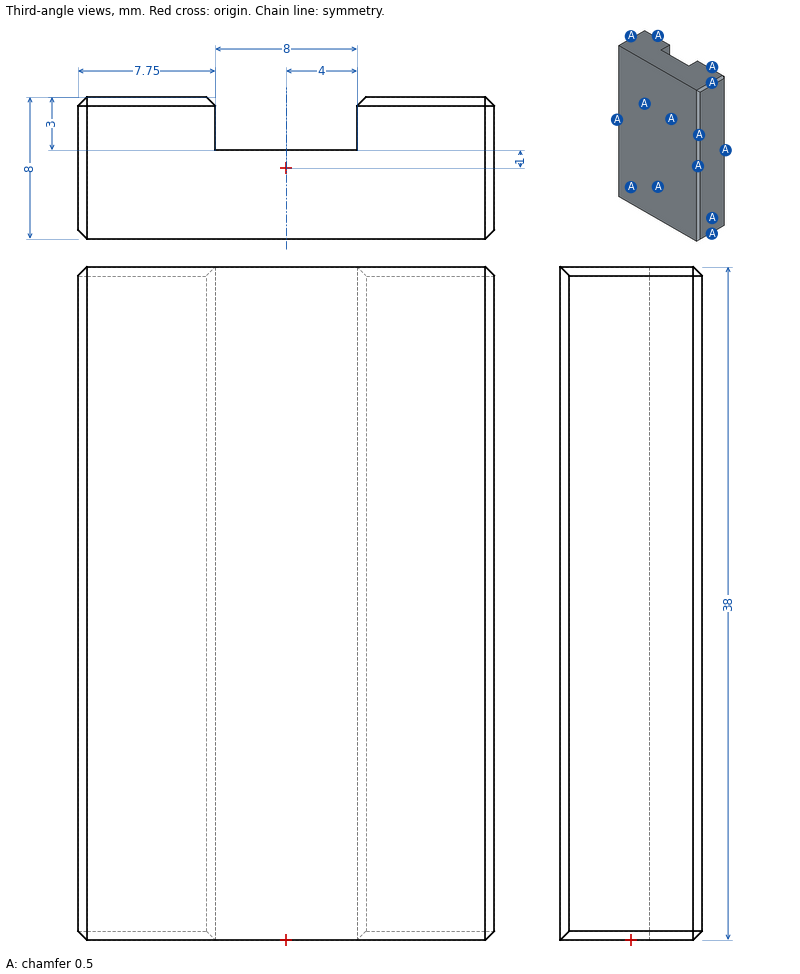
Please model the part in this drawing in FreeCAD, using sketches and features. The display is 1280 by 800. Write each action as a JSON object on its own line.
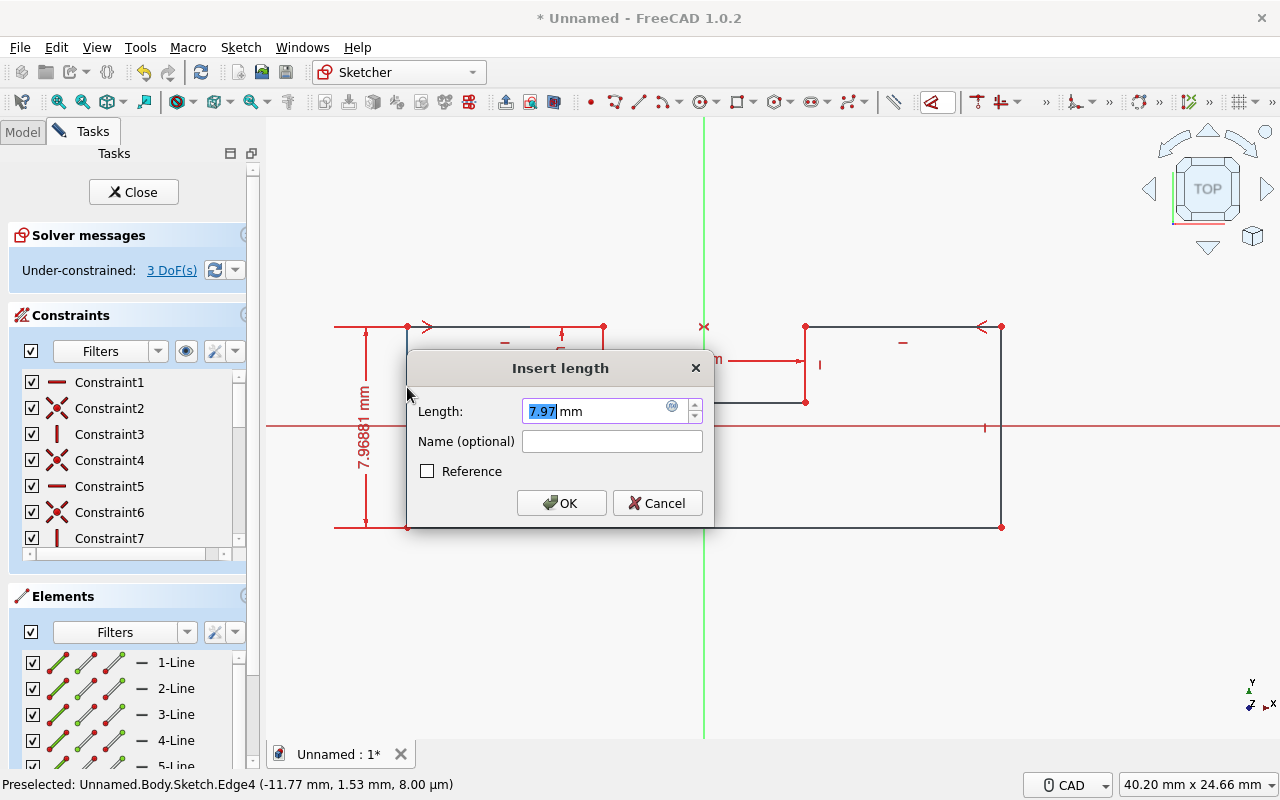
{"action": "type", "text": "8"}
{"action": "key", "text": "Return"}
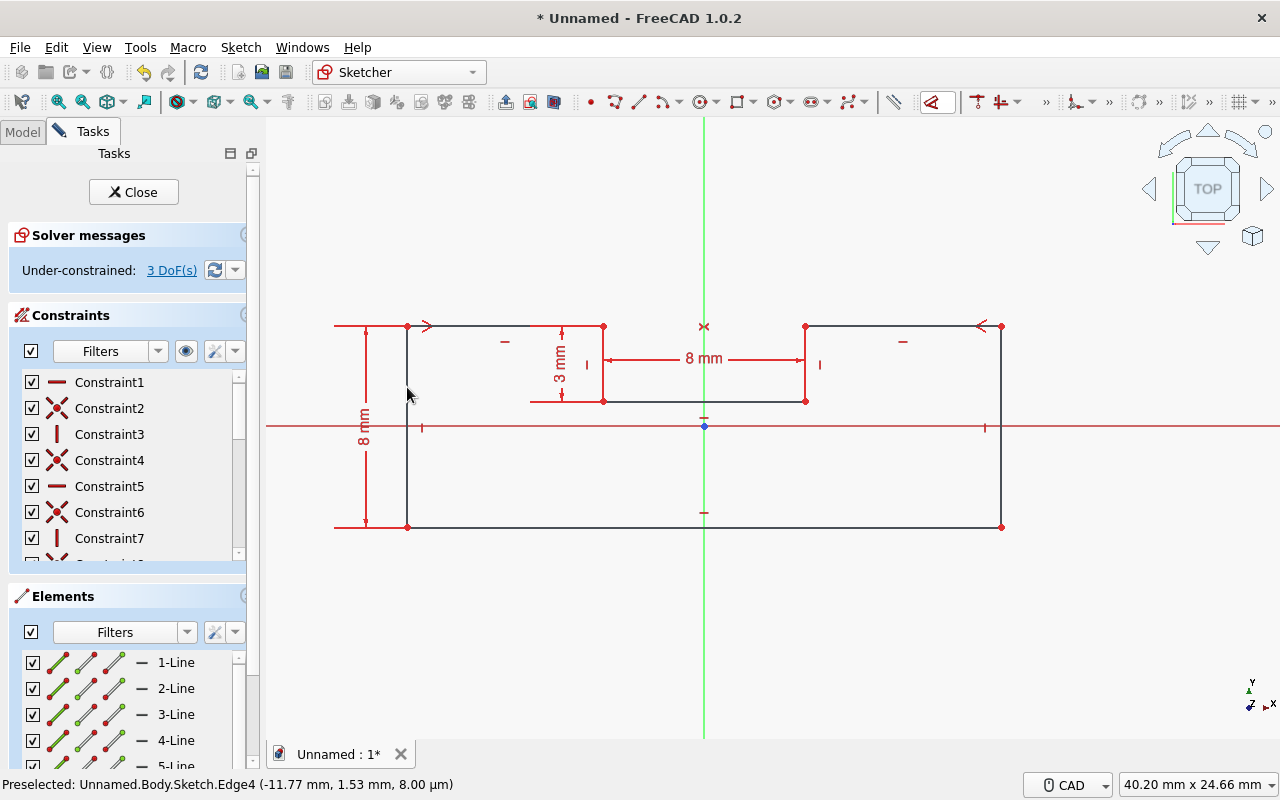
{"action": "left_click", "coordinate": [805, 402]}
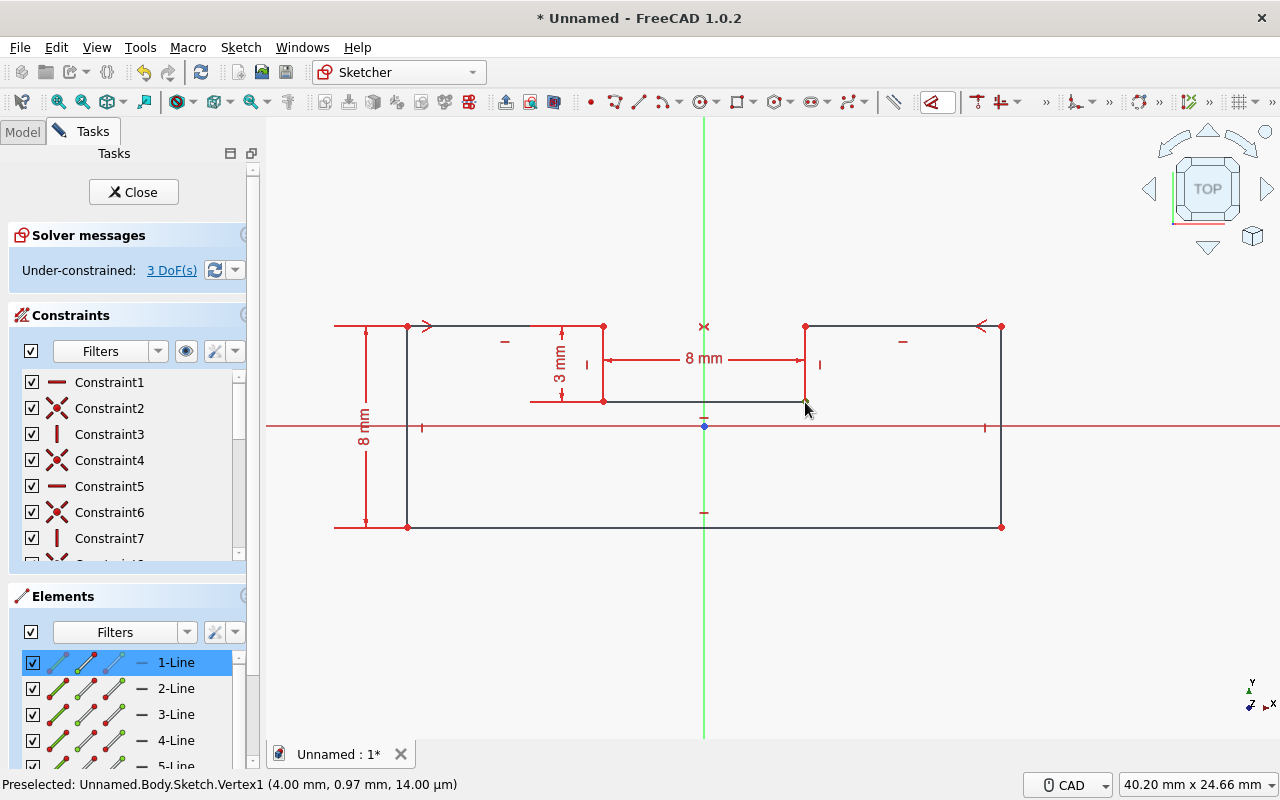
{"action": "key", "text": "l"}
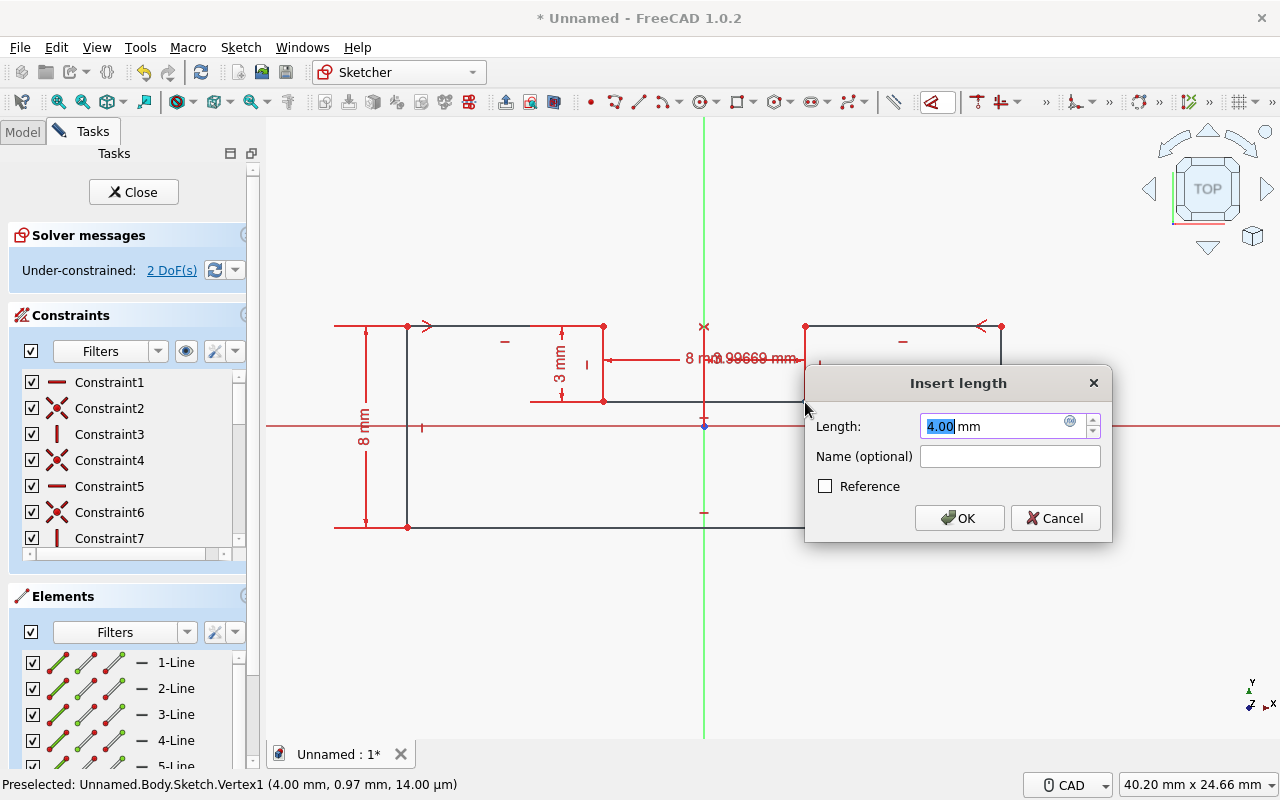
{"action": "type", "text": "4"}
{"action": "key", "text": "Return"}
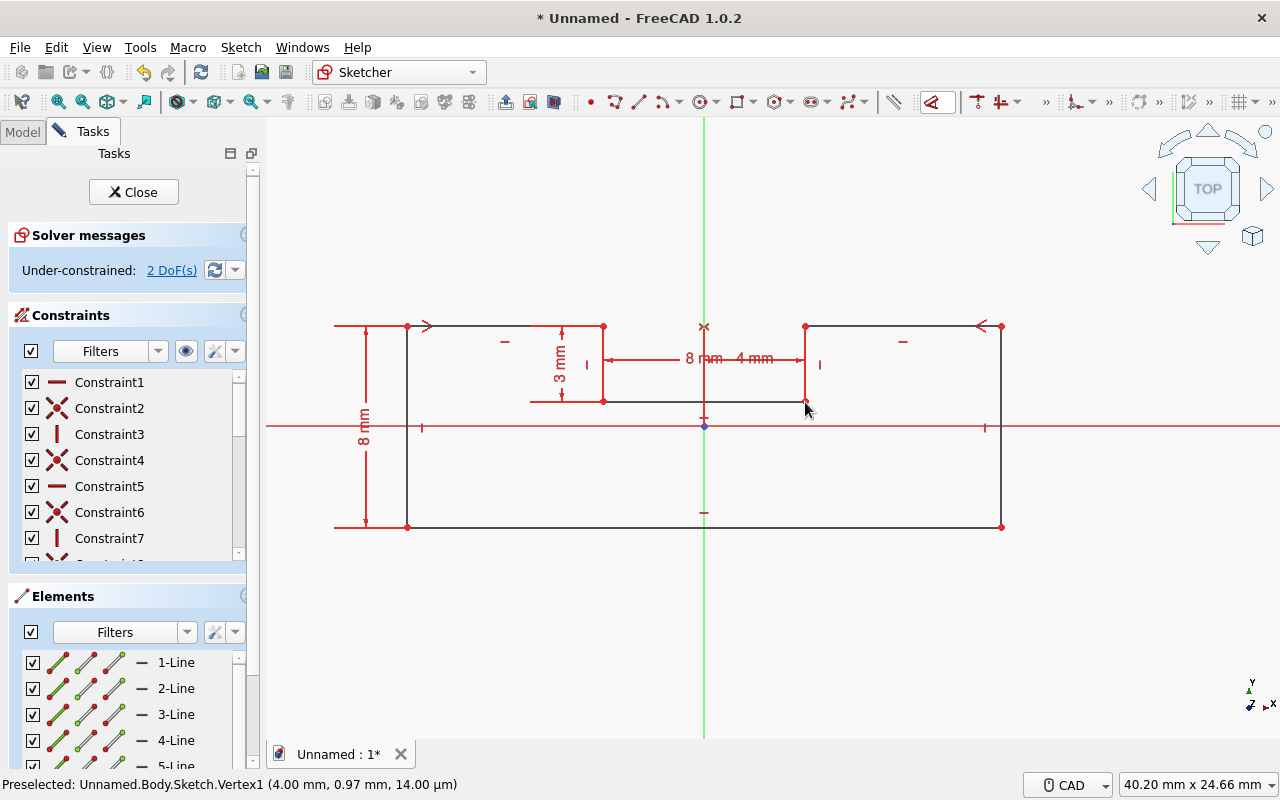
{"action": "scroll", "coordinate": [805, 402], "scroll_direction": "up", "scroll_amount": 3}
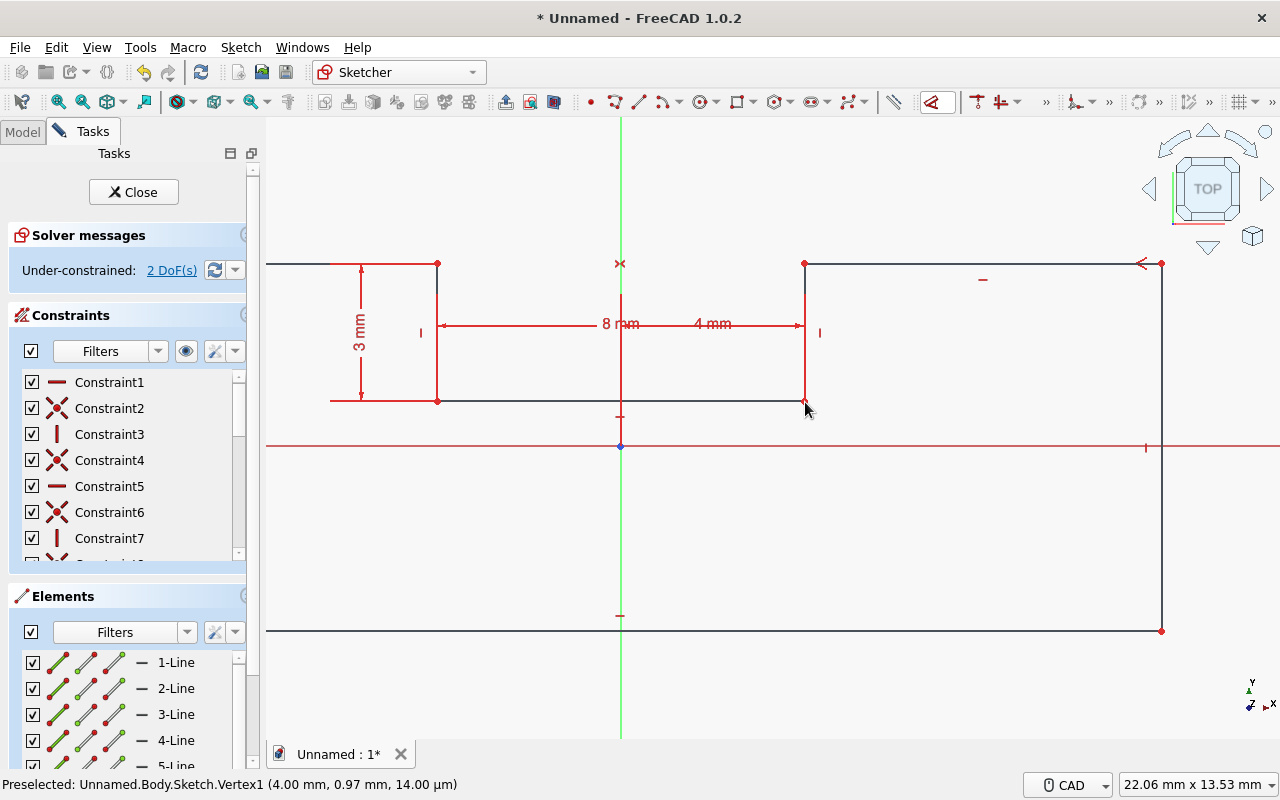
{"action": "left_click", "coordinate": [805, 401]}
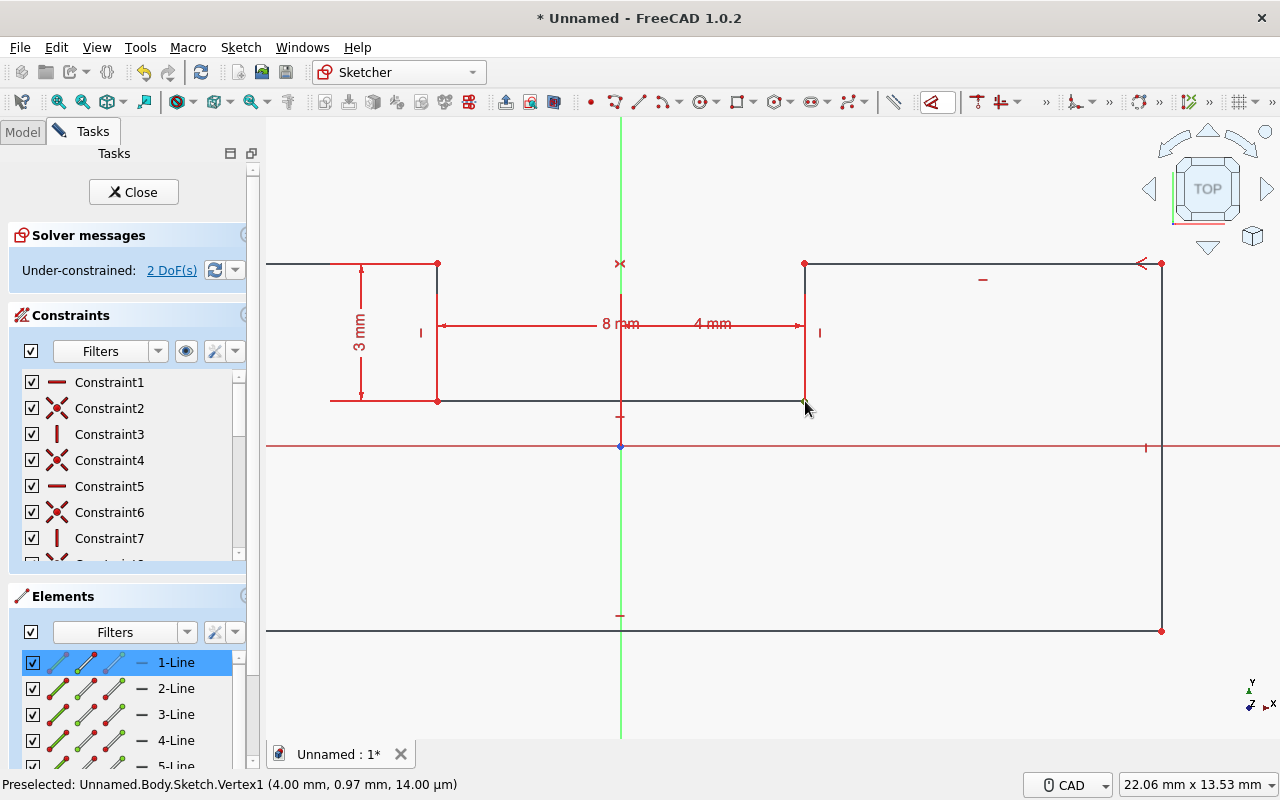
{"action": "key", "text": "i"}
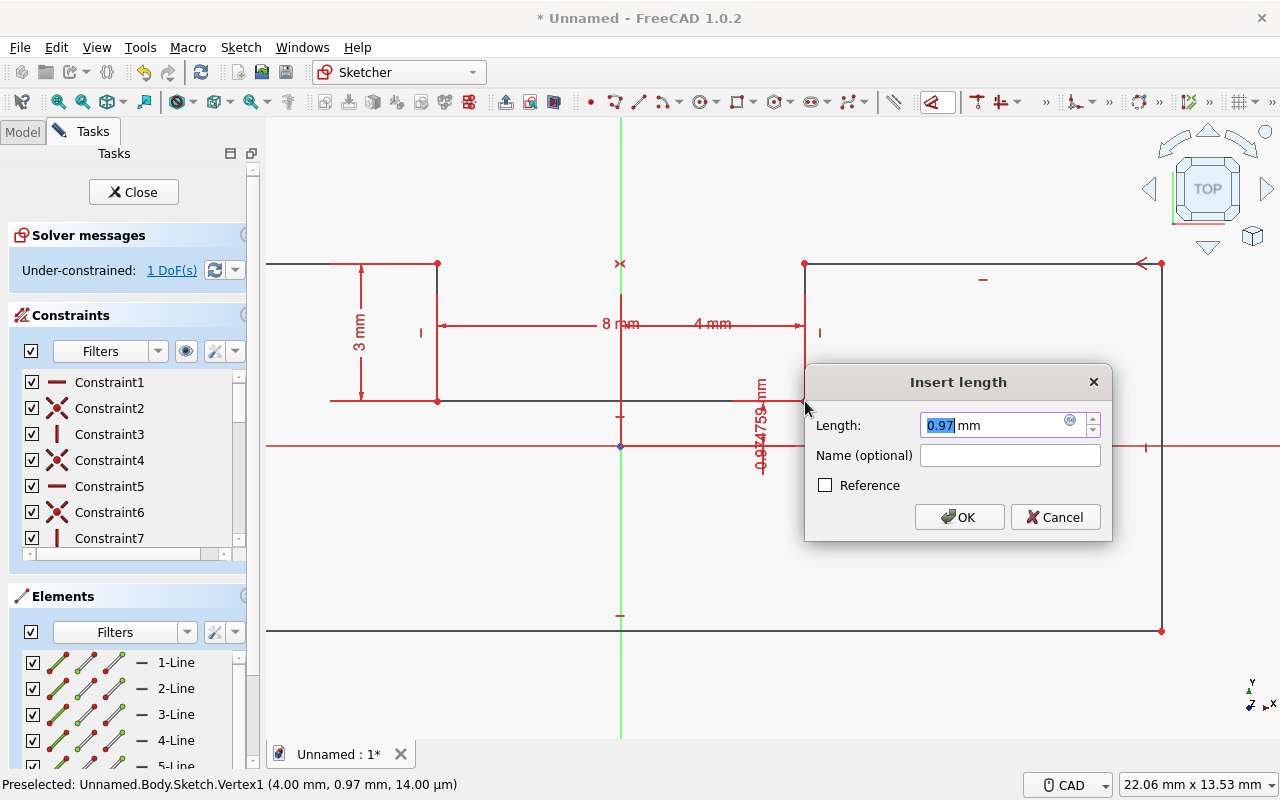
{"action": "type", "text": "1"}
{"action": "key", "text": "Return"}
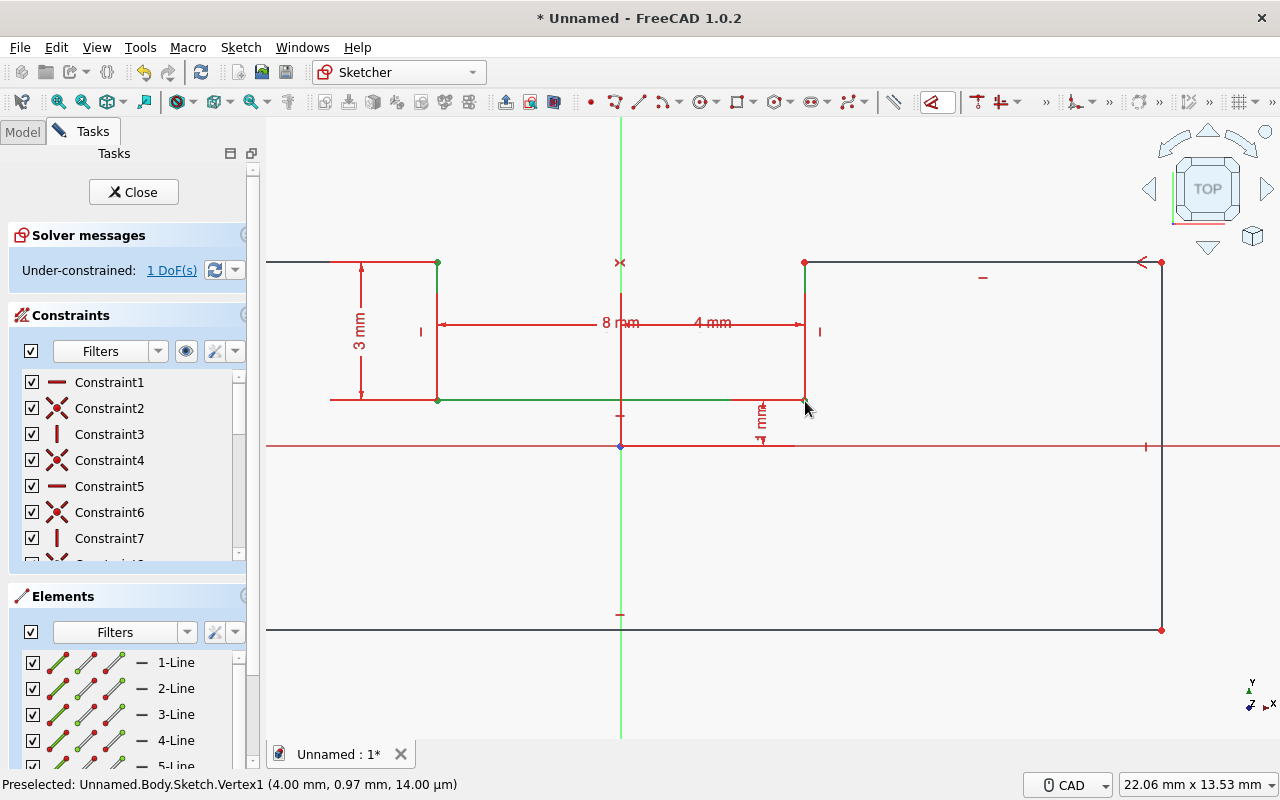
{"action": "left_click", "coordinate": [330, 262]}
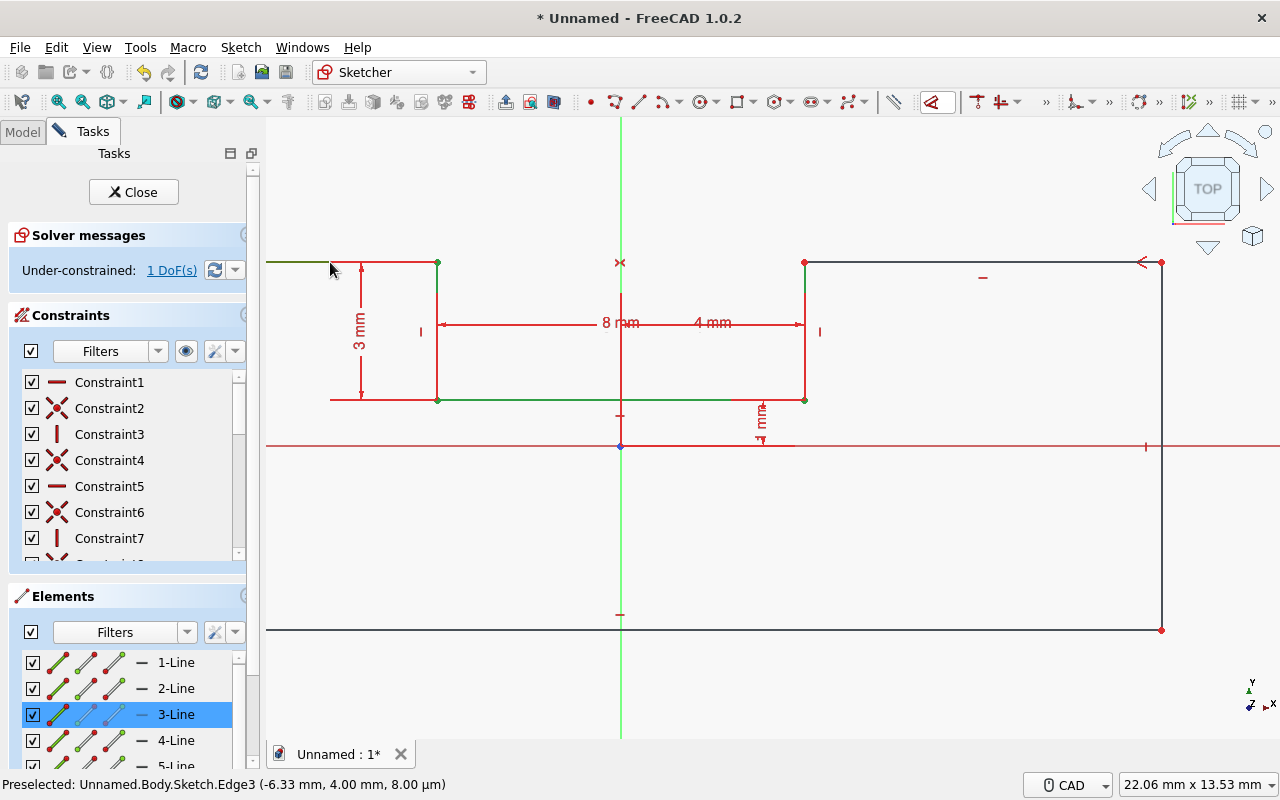
{"action": "key", "text": "l"}